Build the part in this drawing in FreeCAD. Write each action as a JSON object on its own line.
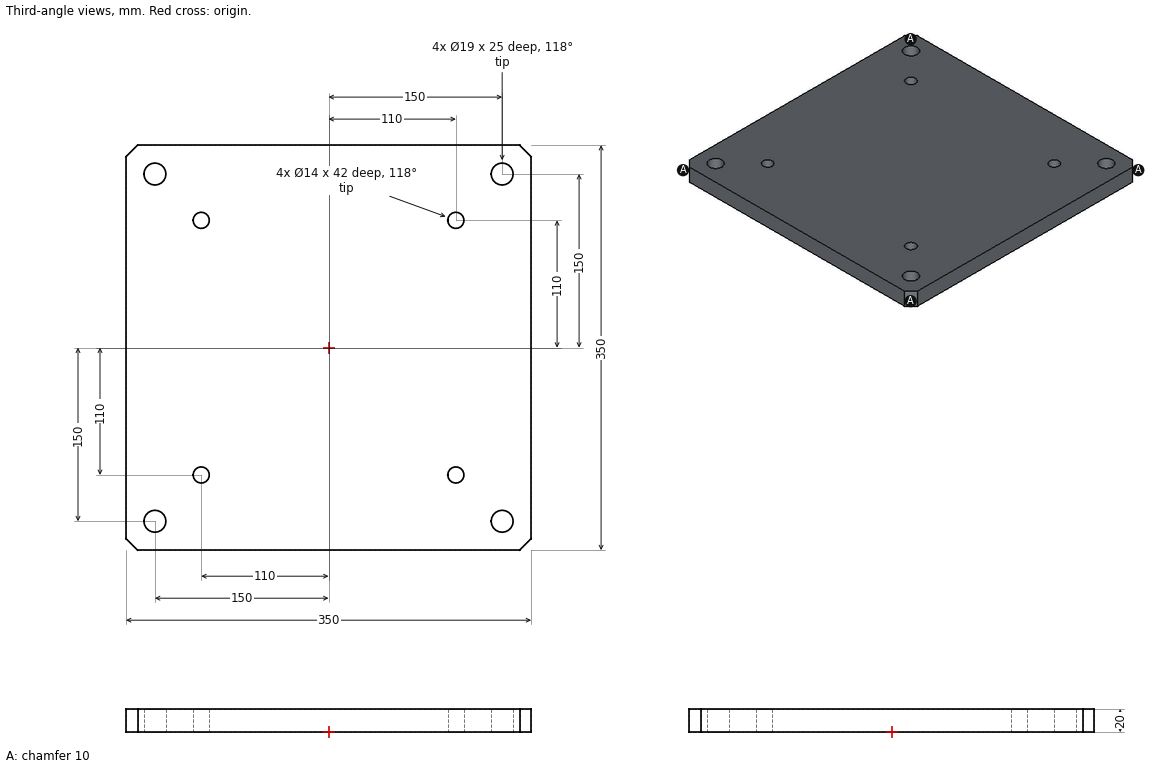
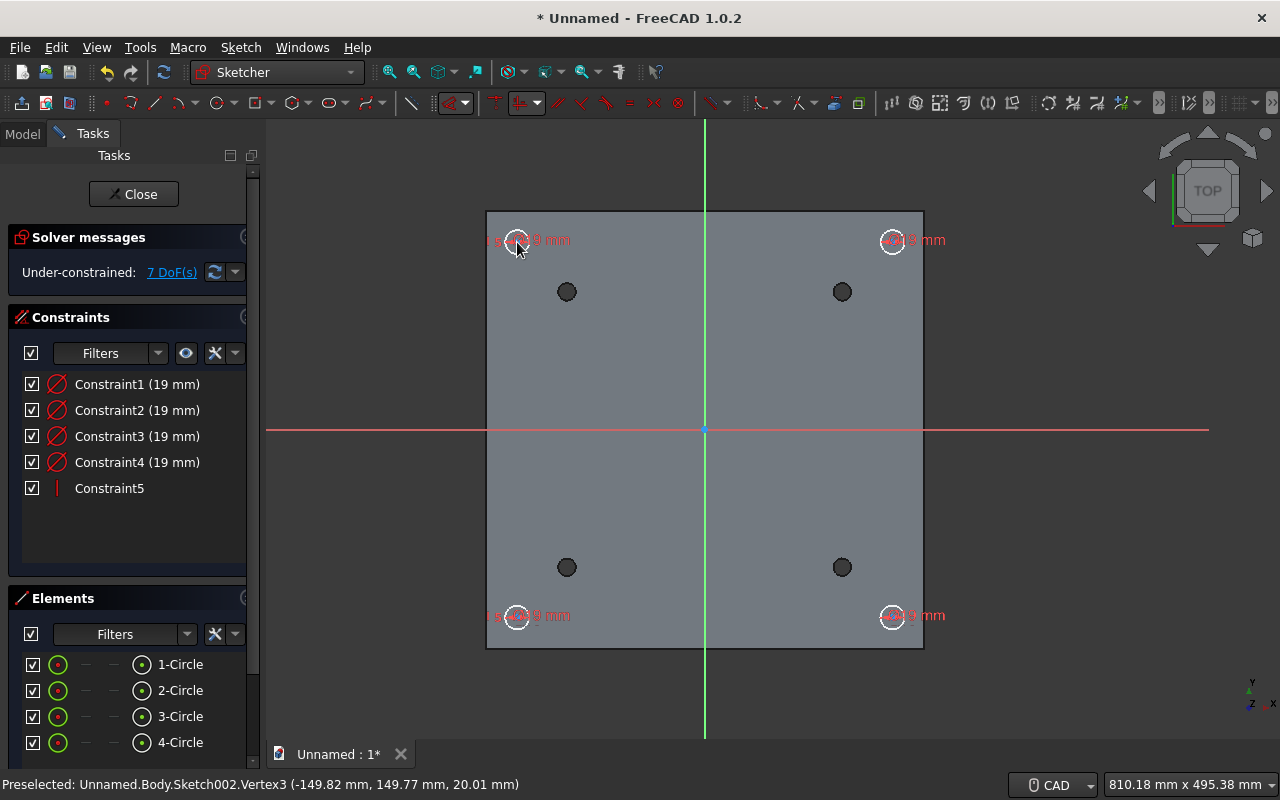
{"action": "left_click", "coordinate": [893, 242]}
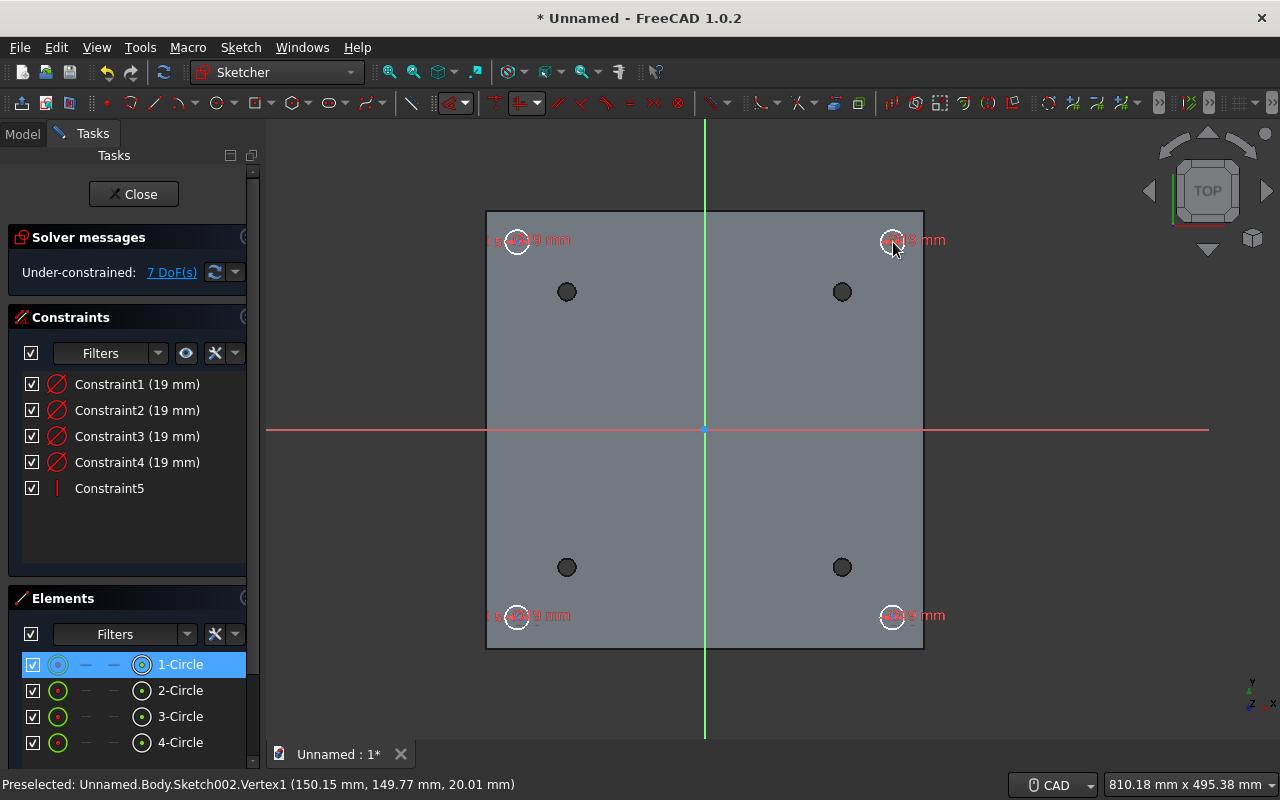
{"action": "left_click", "coordinate": [517, 242]}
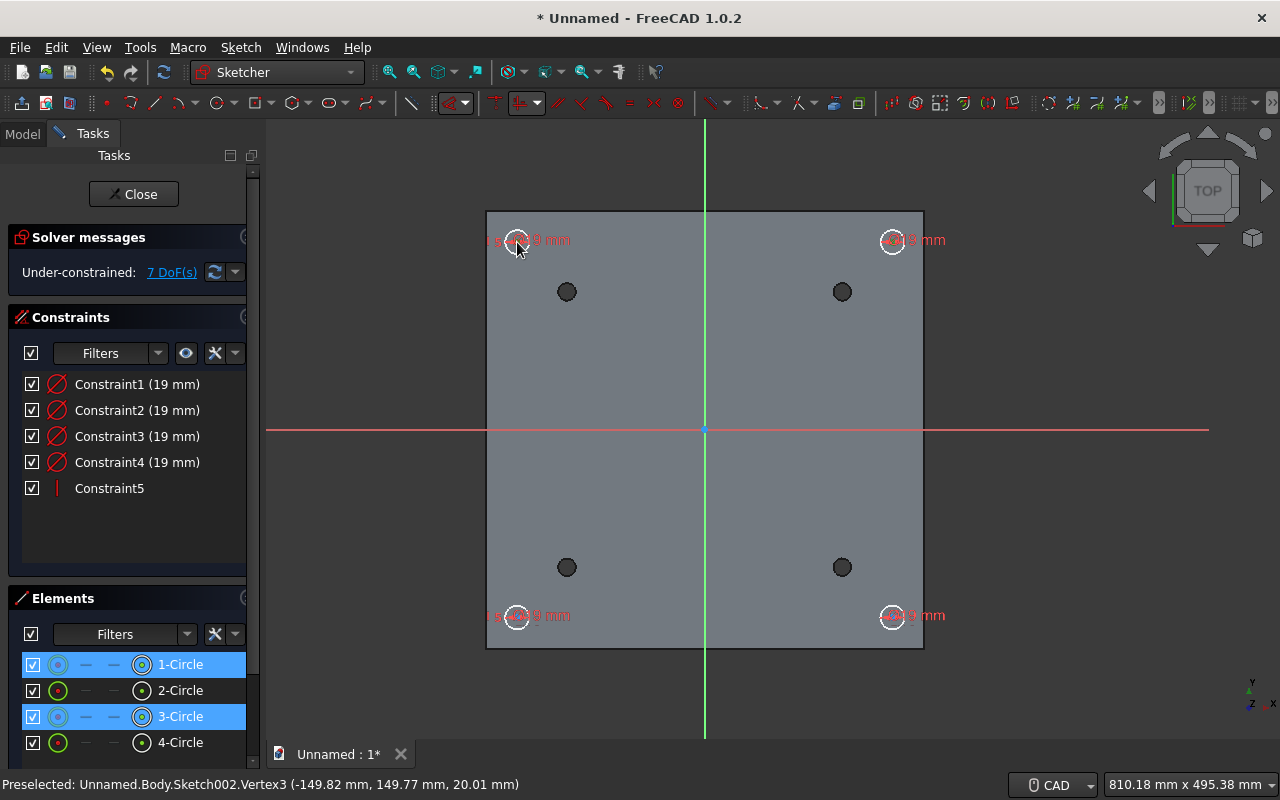
{"action": "left_click", "coordinate": [540, 104]}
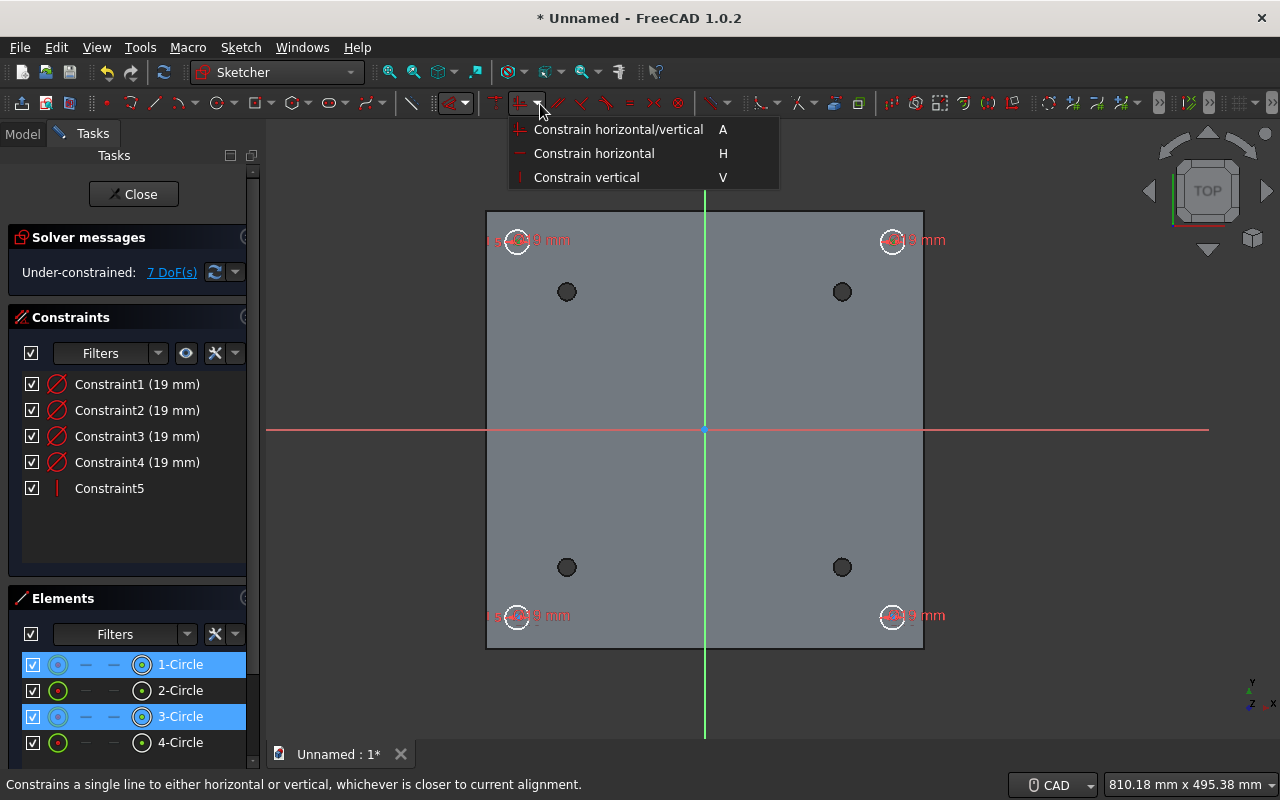
{"action": "left_click", "coordinate": [644, 153]}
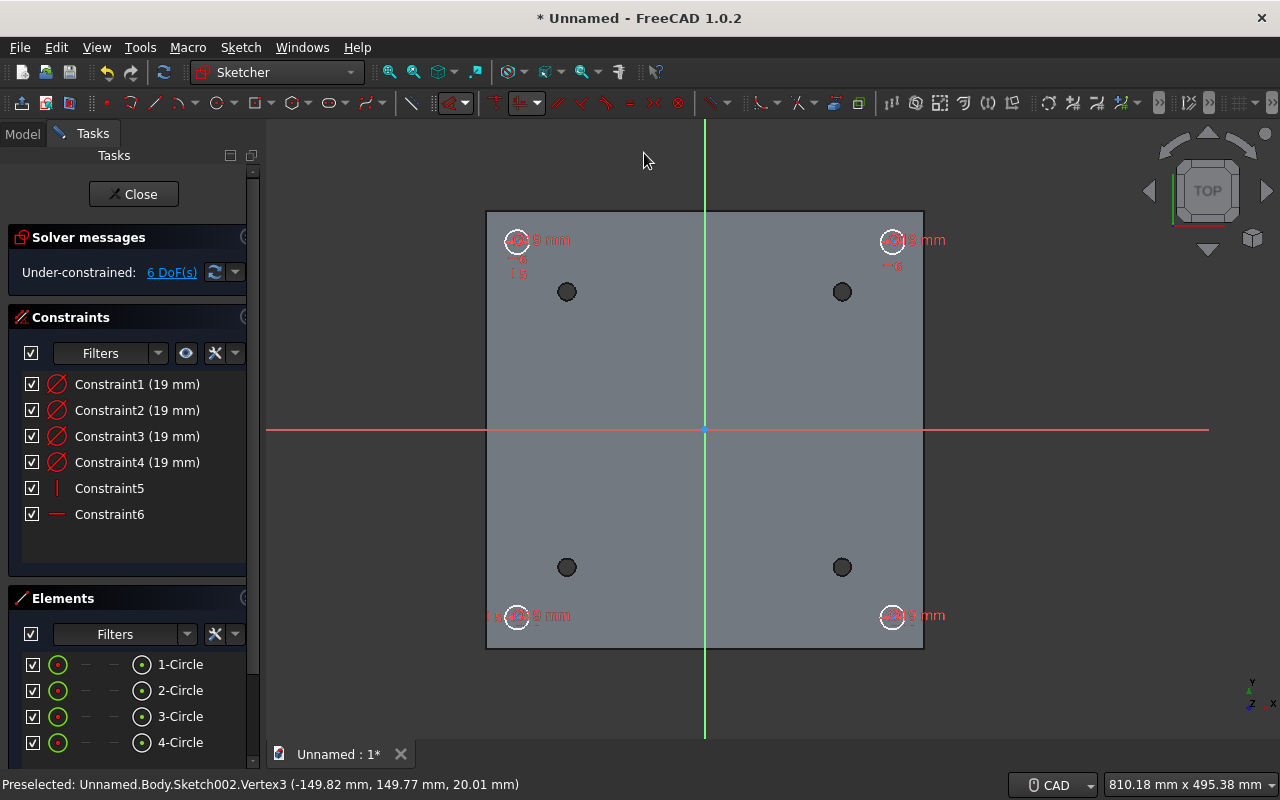
{"action": "left_click", "coordinate": [893, 242]}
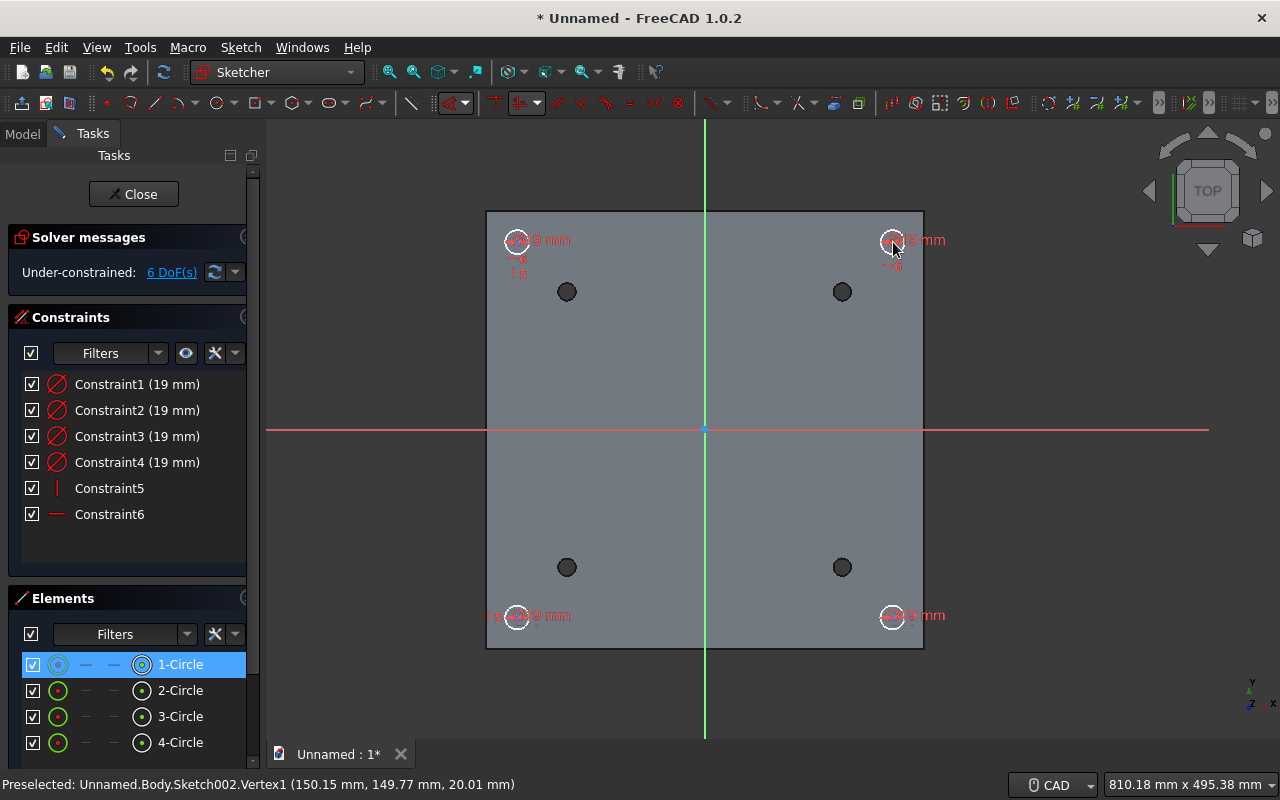
{"action": "left_click", "coordinate": [892, 618]}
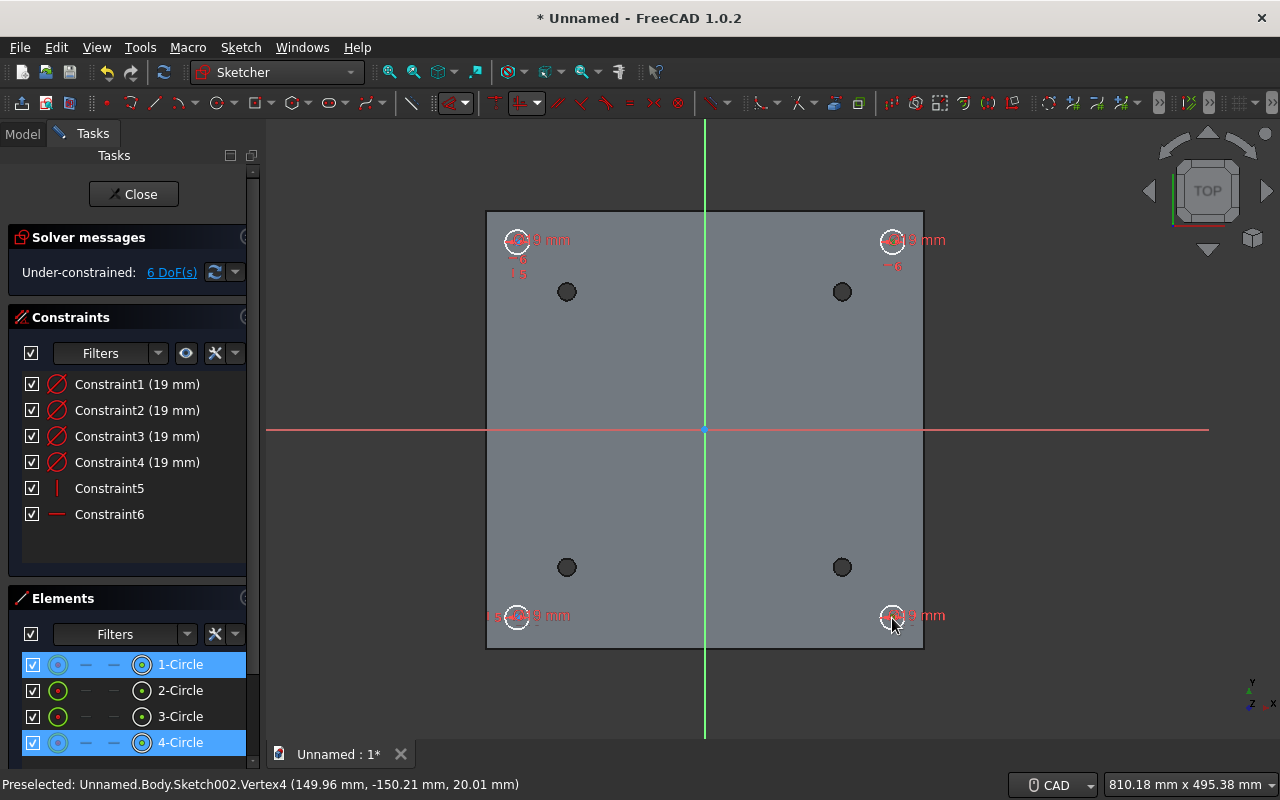
{"action": "left_click", "coordinate": [540, 104]}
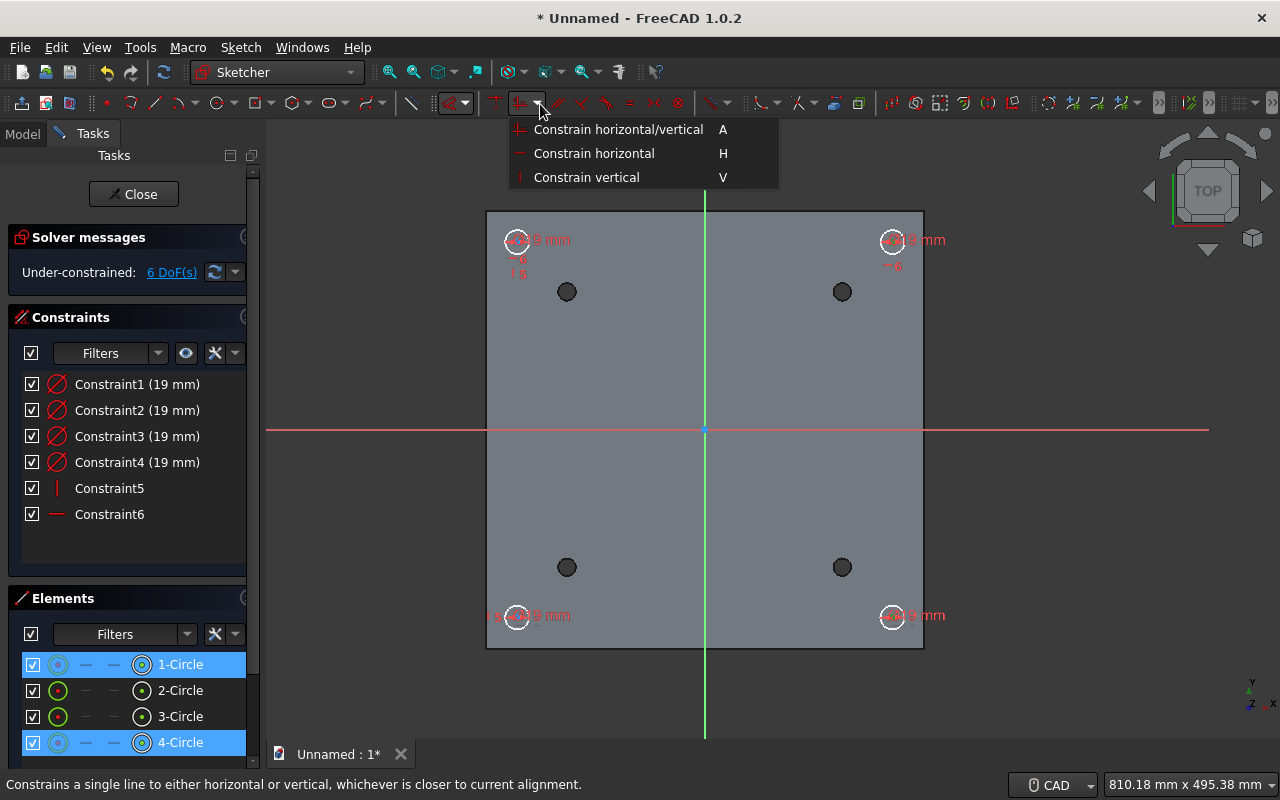
{"action": "left_click", "coordinate": [644, 177]}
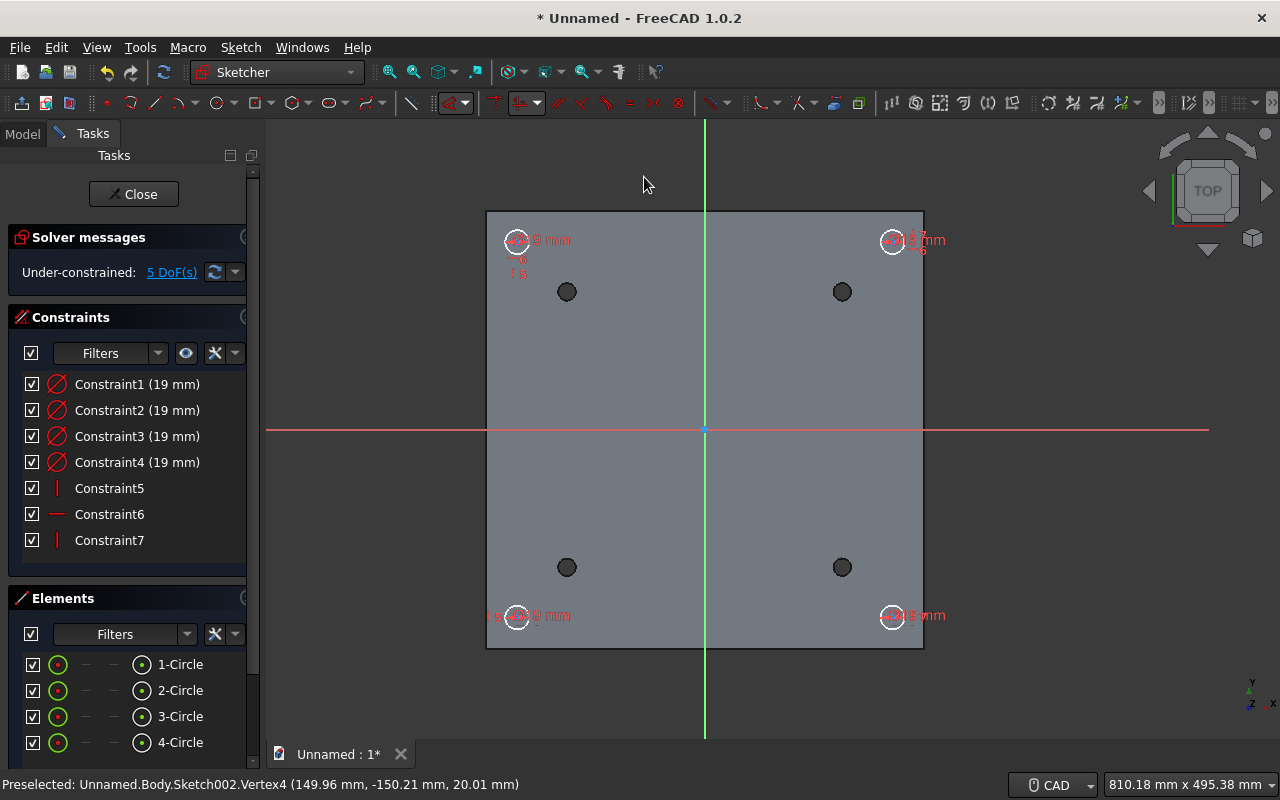
{"action": "left_click", "coordinate": [517, 618]}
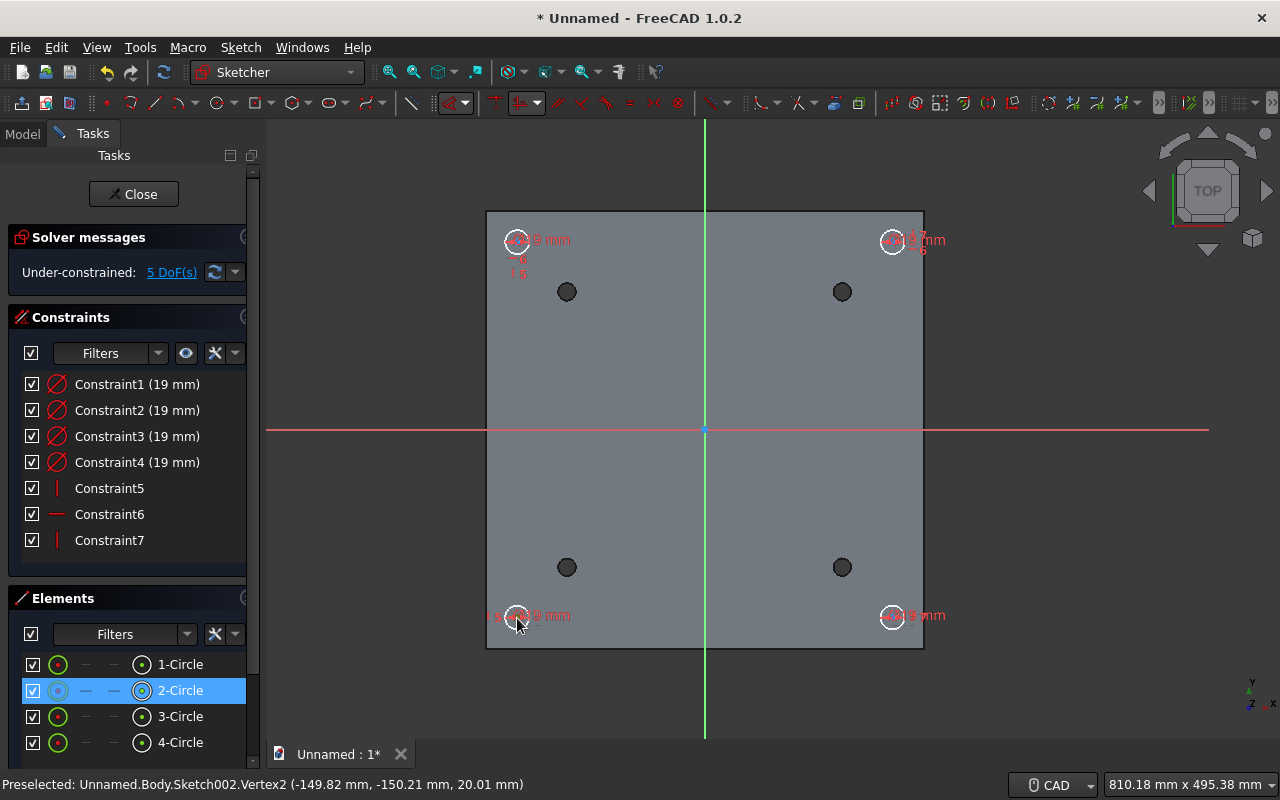
{"action": "left_click", "coordinate": [893, 618]}